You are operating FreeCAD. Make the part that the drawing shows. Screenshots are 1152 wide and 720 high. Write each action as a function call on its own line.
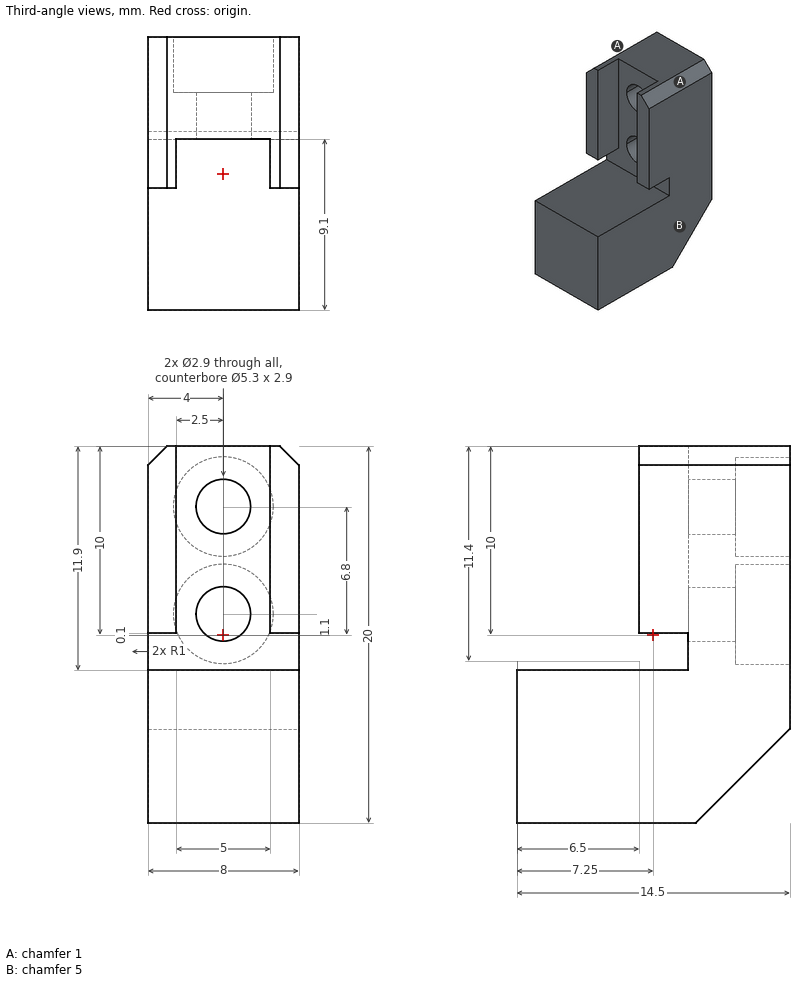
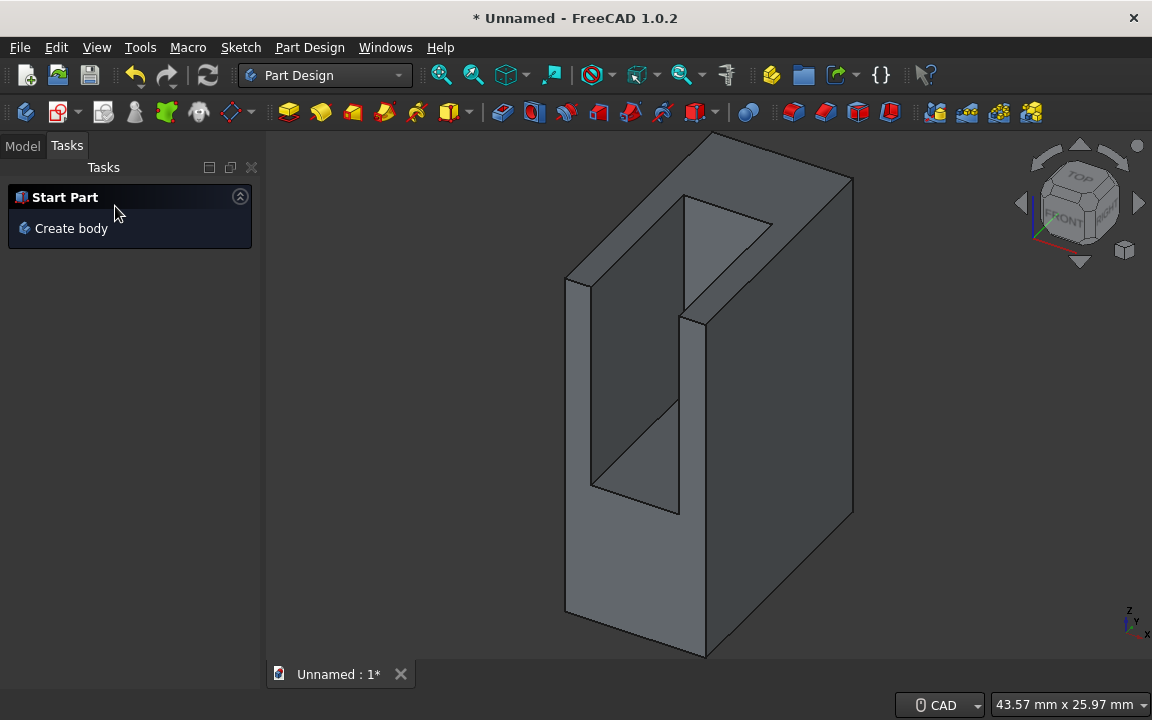
key(4)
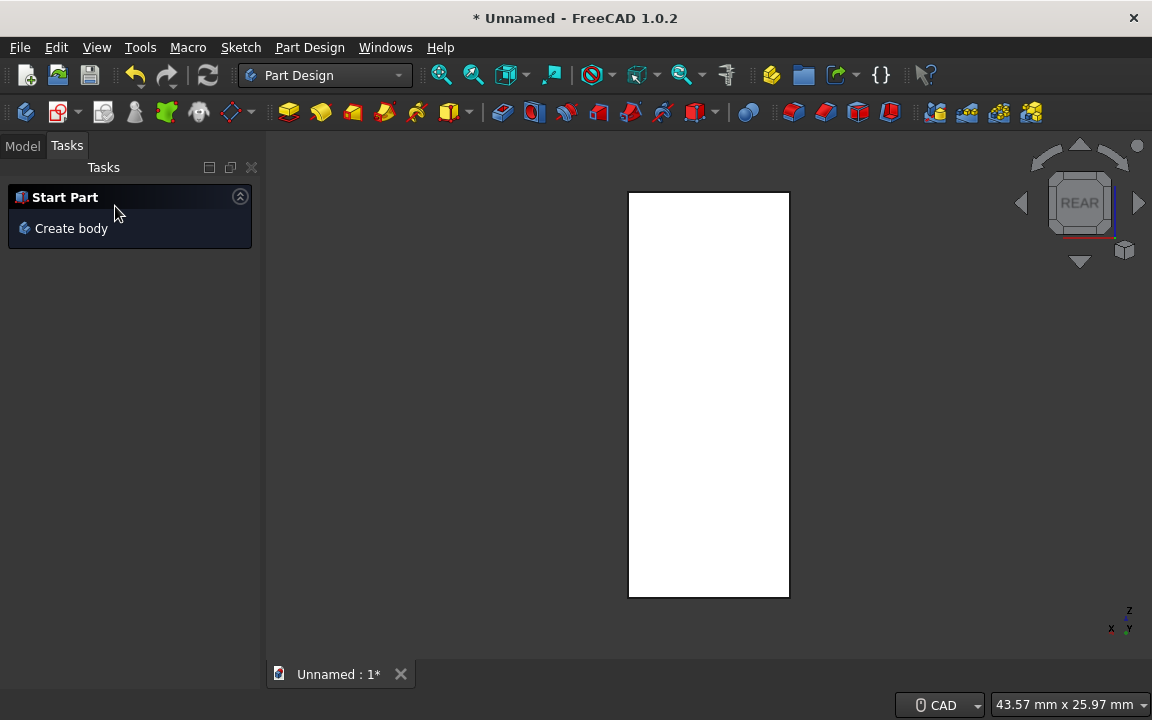
click(709, 278)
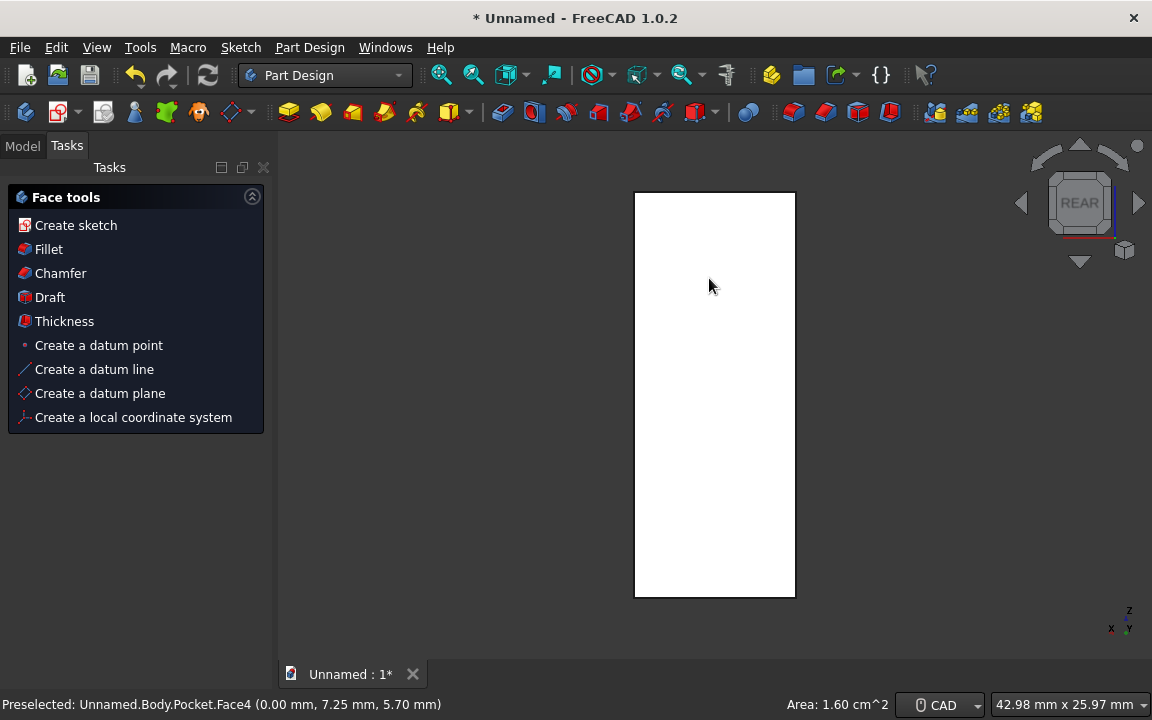
click(58, 112)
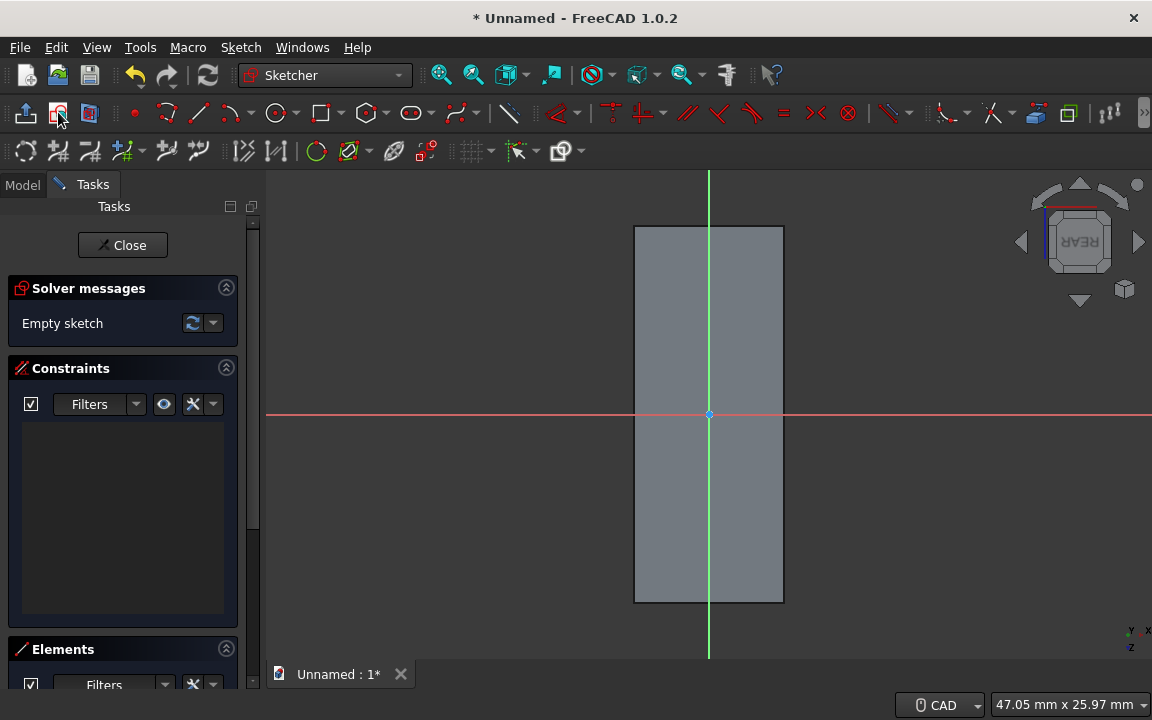
scroll(792, 579, up, 3)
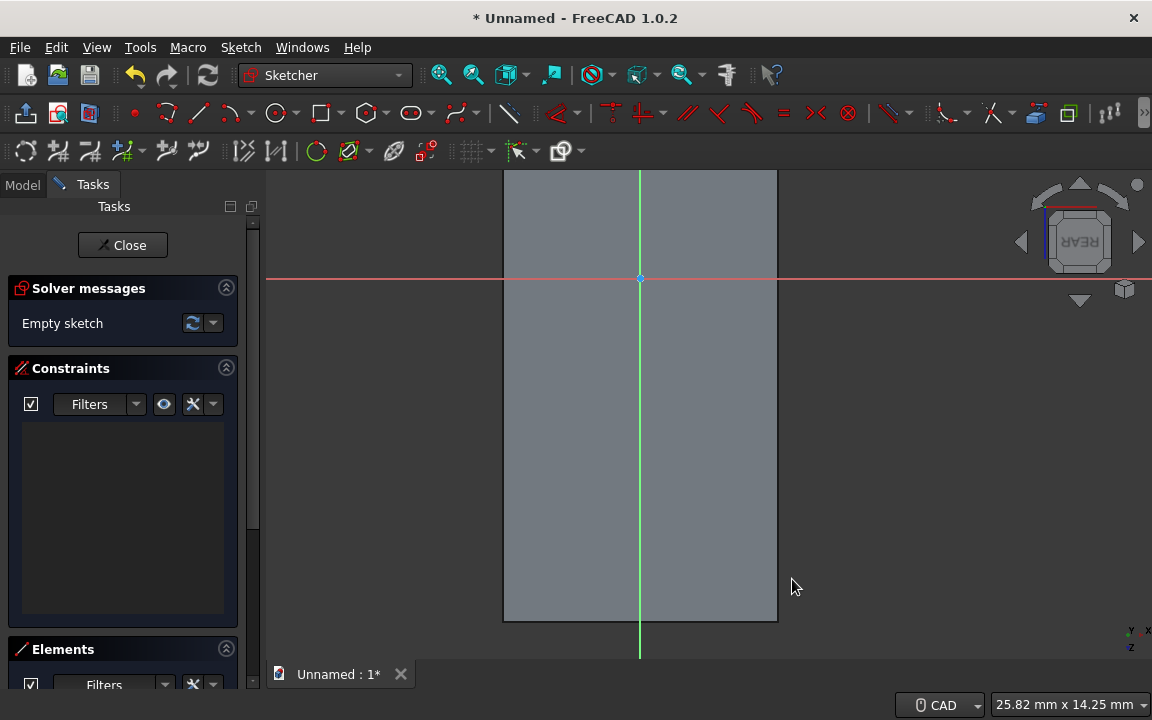
key(g)
key(c)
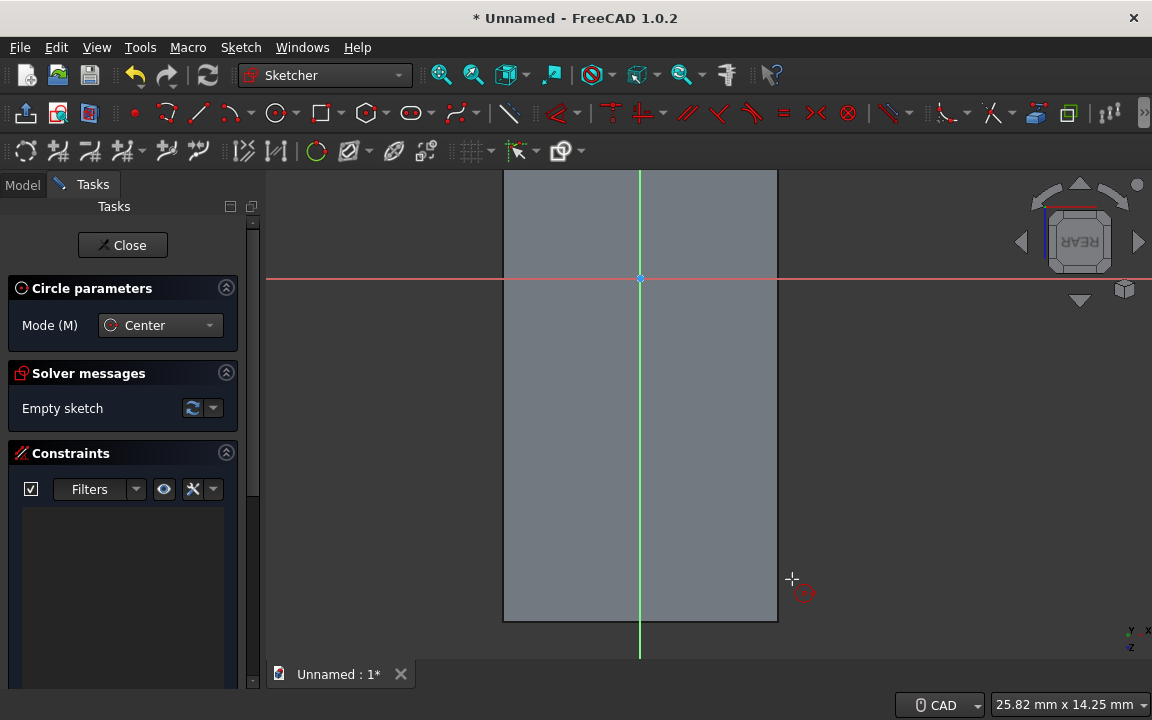
click(640, 512)
click(675, 477)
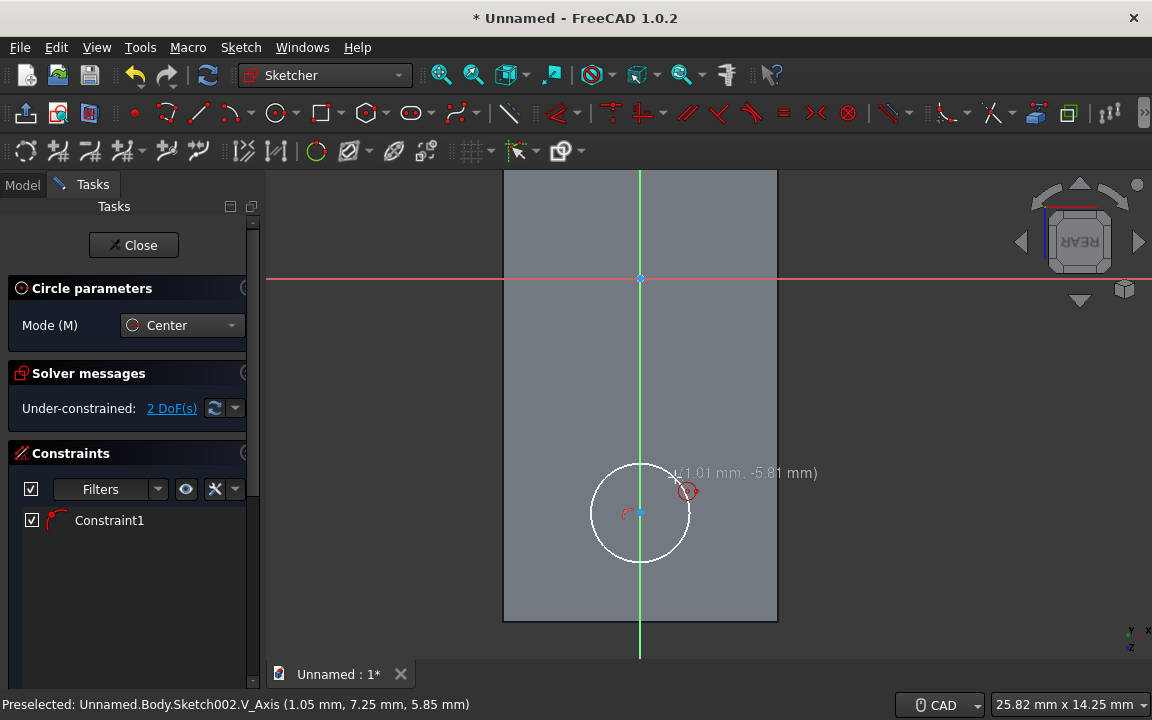
click(640, 316)
click(675, 352)
key(Escape)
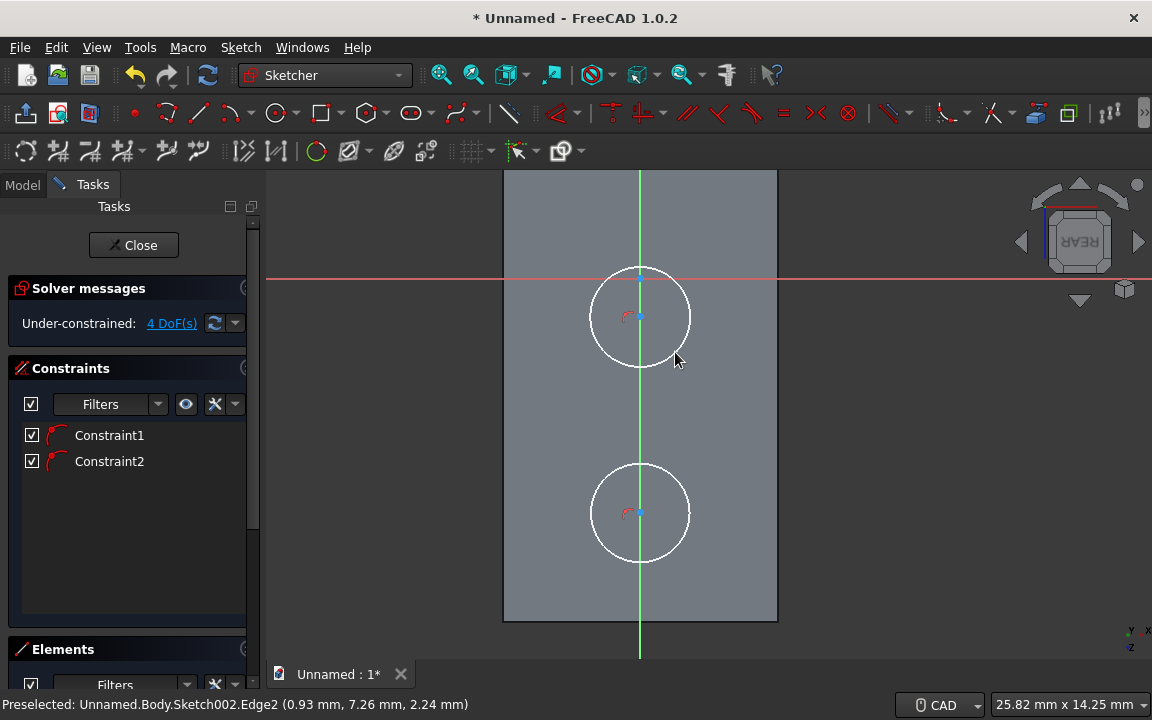
click(675, 478)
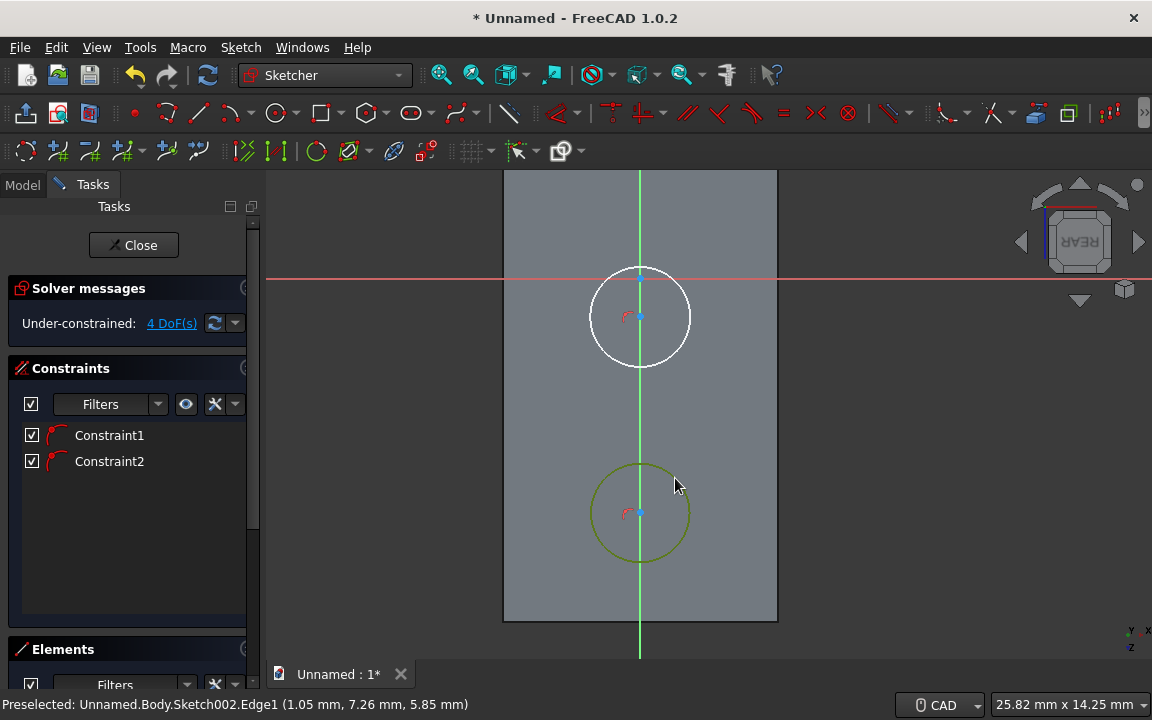
click(676, 282)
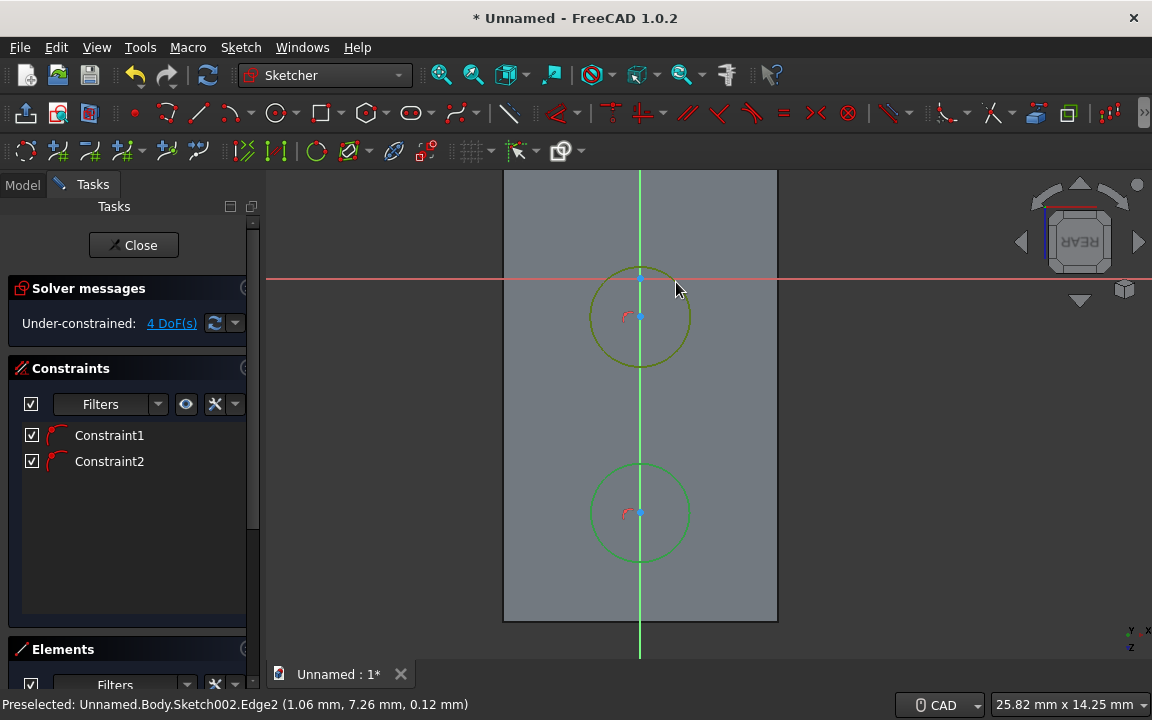
key(e)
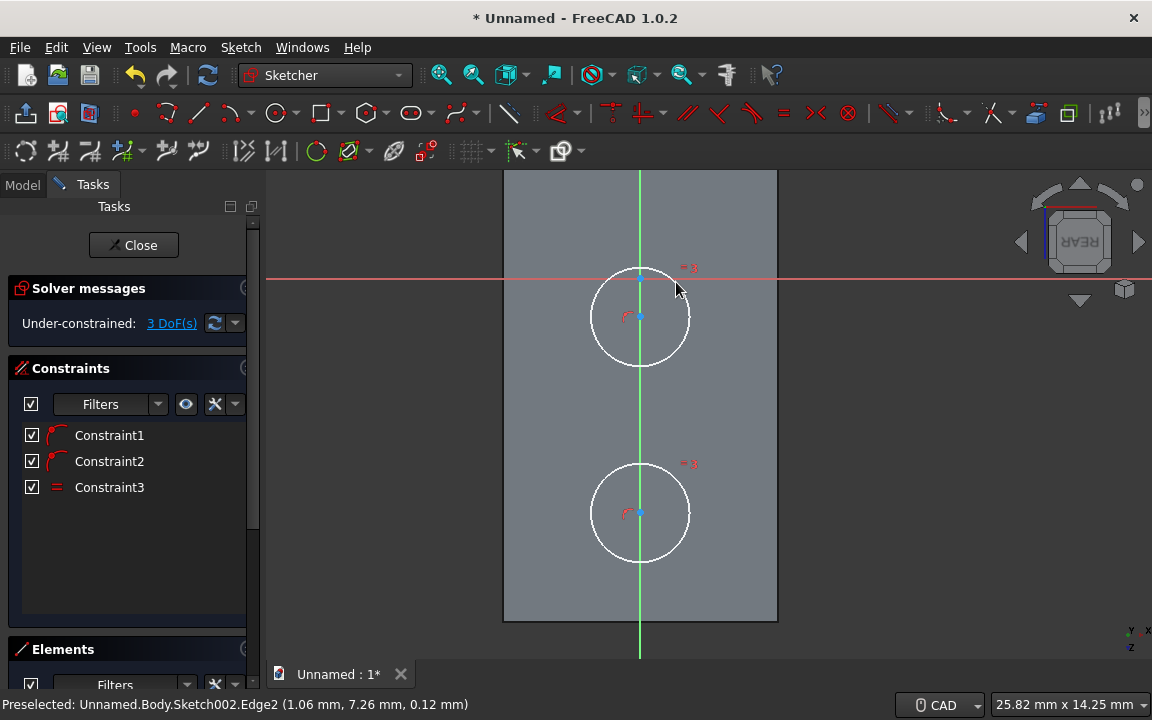
click(556, 114)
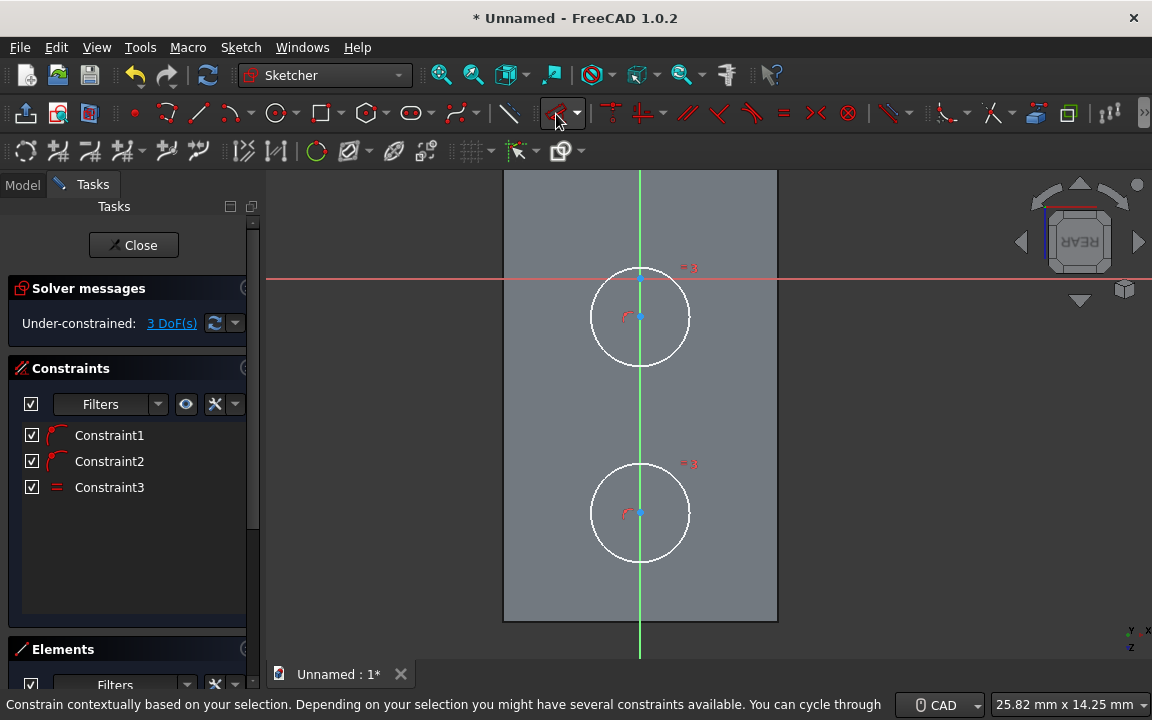
click(675, 478)
click(698, 455)